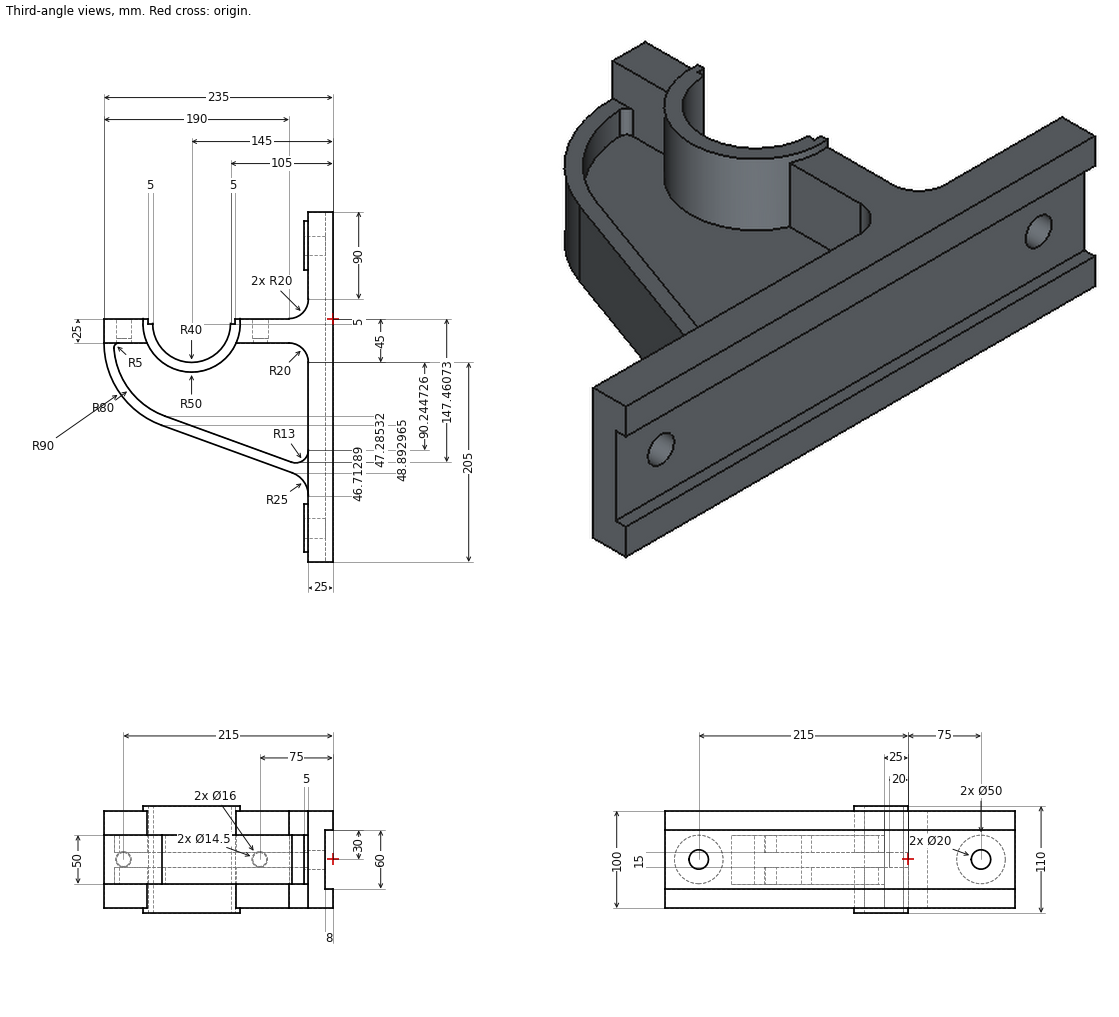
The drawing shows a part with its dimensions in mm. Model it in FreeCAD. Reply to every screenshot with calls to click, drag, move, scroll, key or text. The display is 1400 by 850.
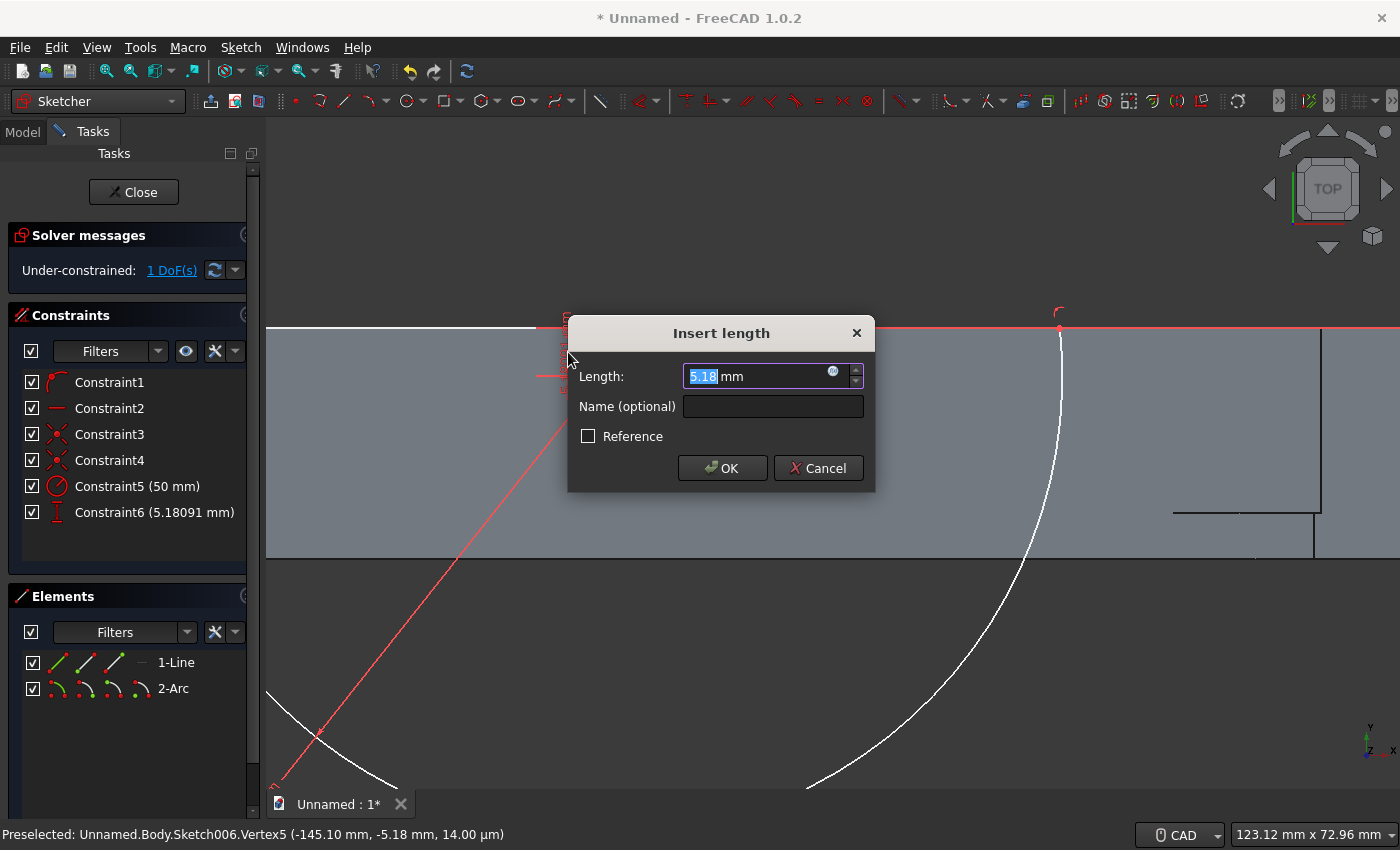
text(5)
key(Return)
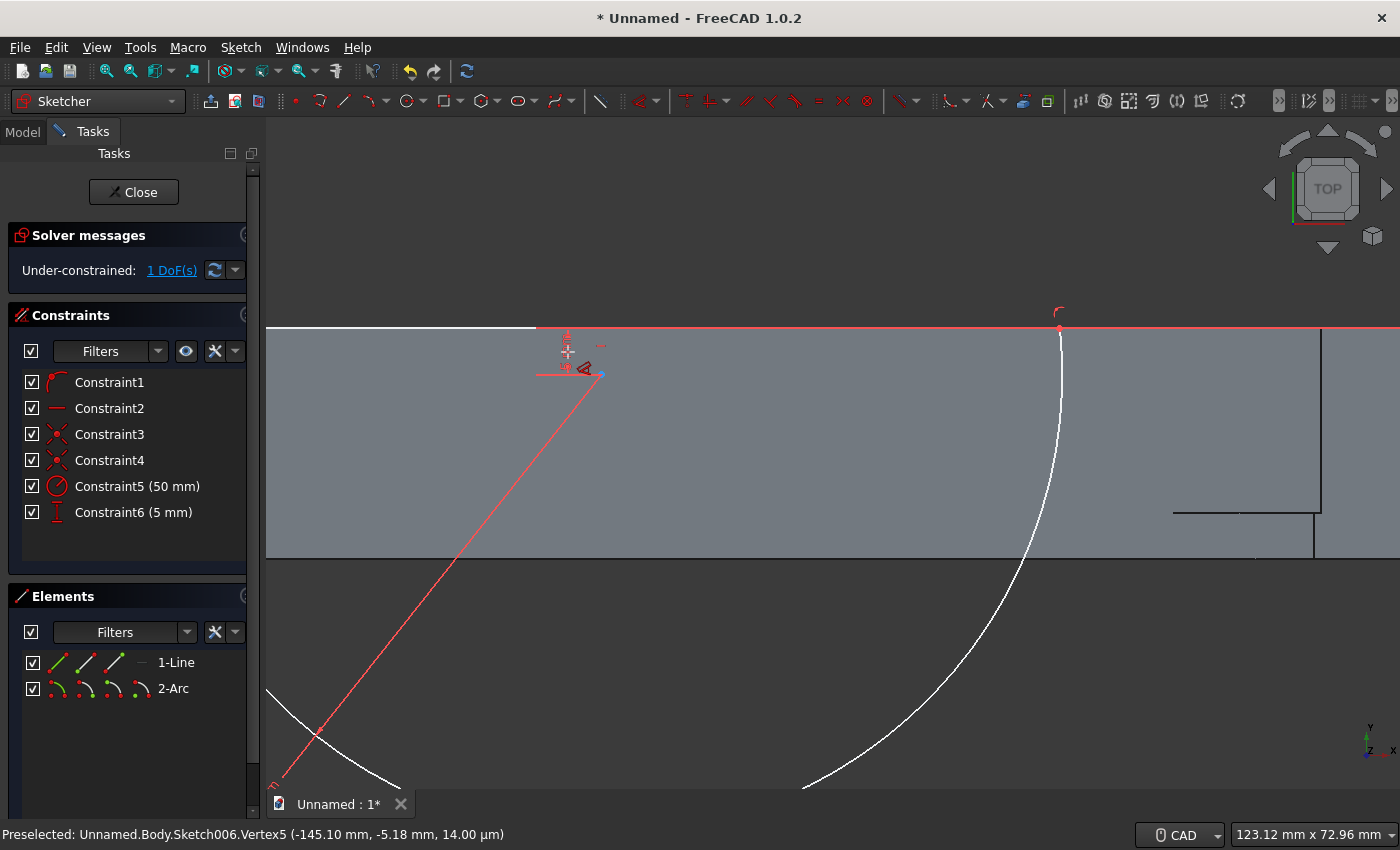
click(602, 375)
click(918, 294)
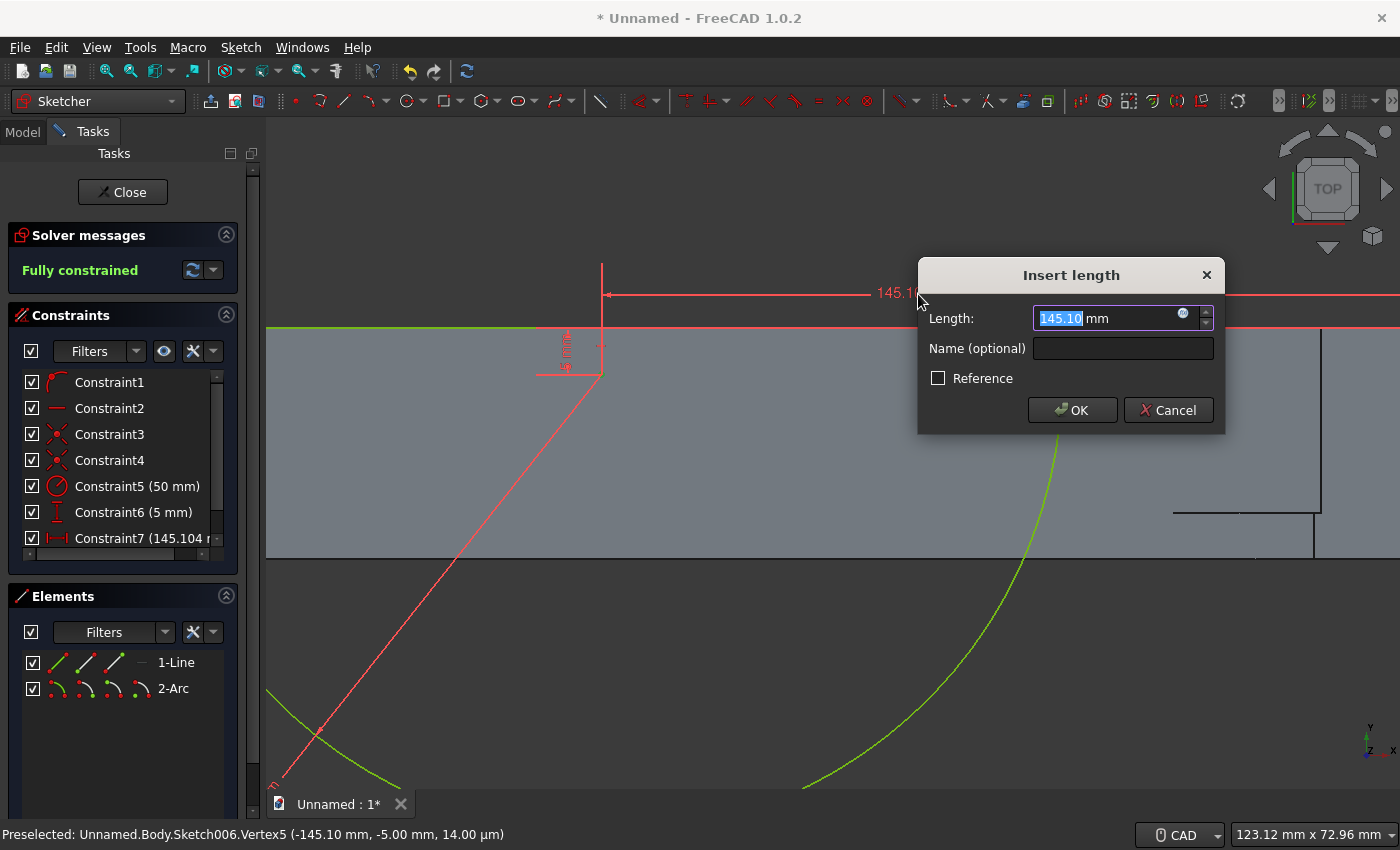
text(145)
key(Return)
key(Escape)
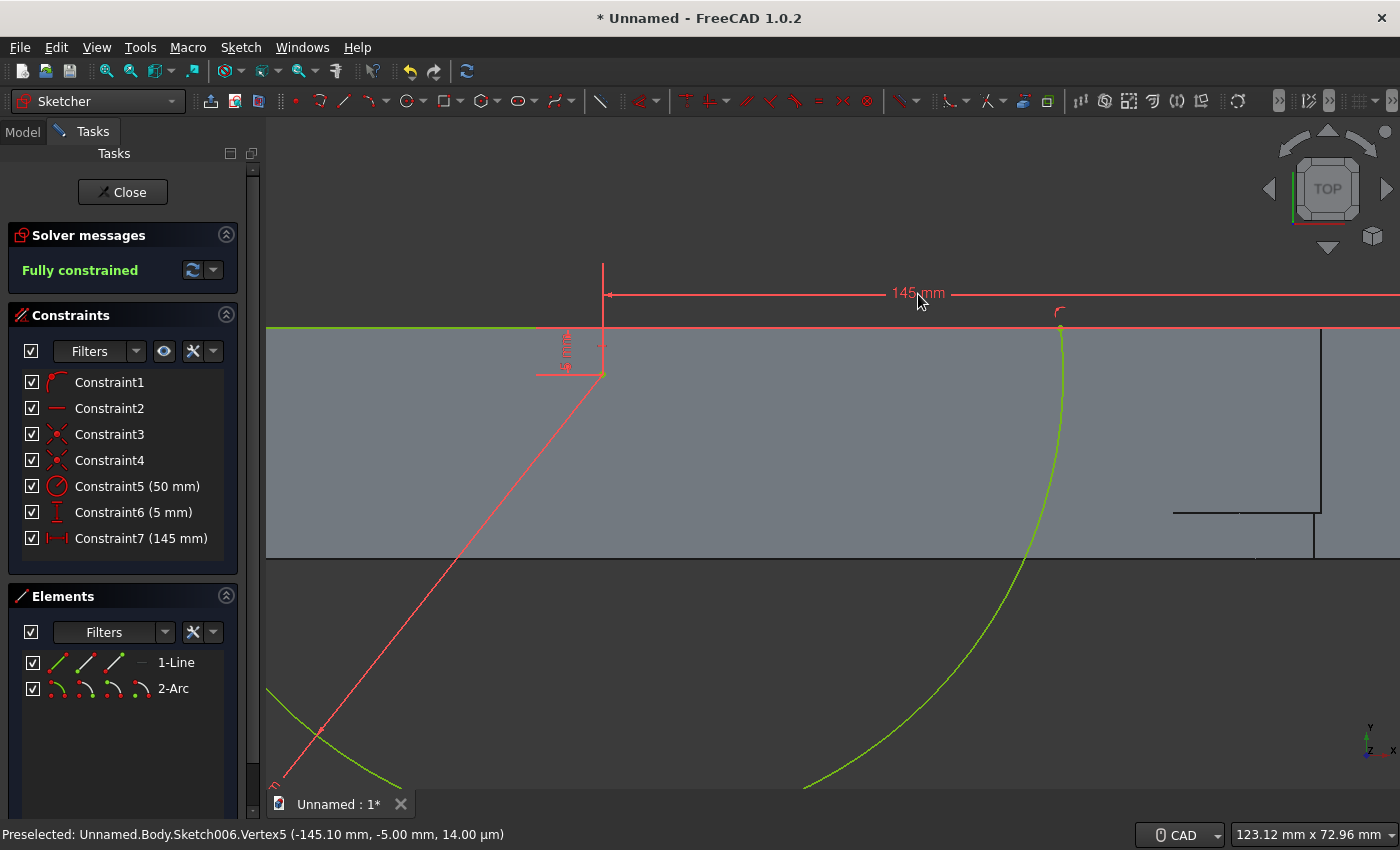
click(123, 192)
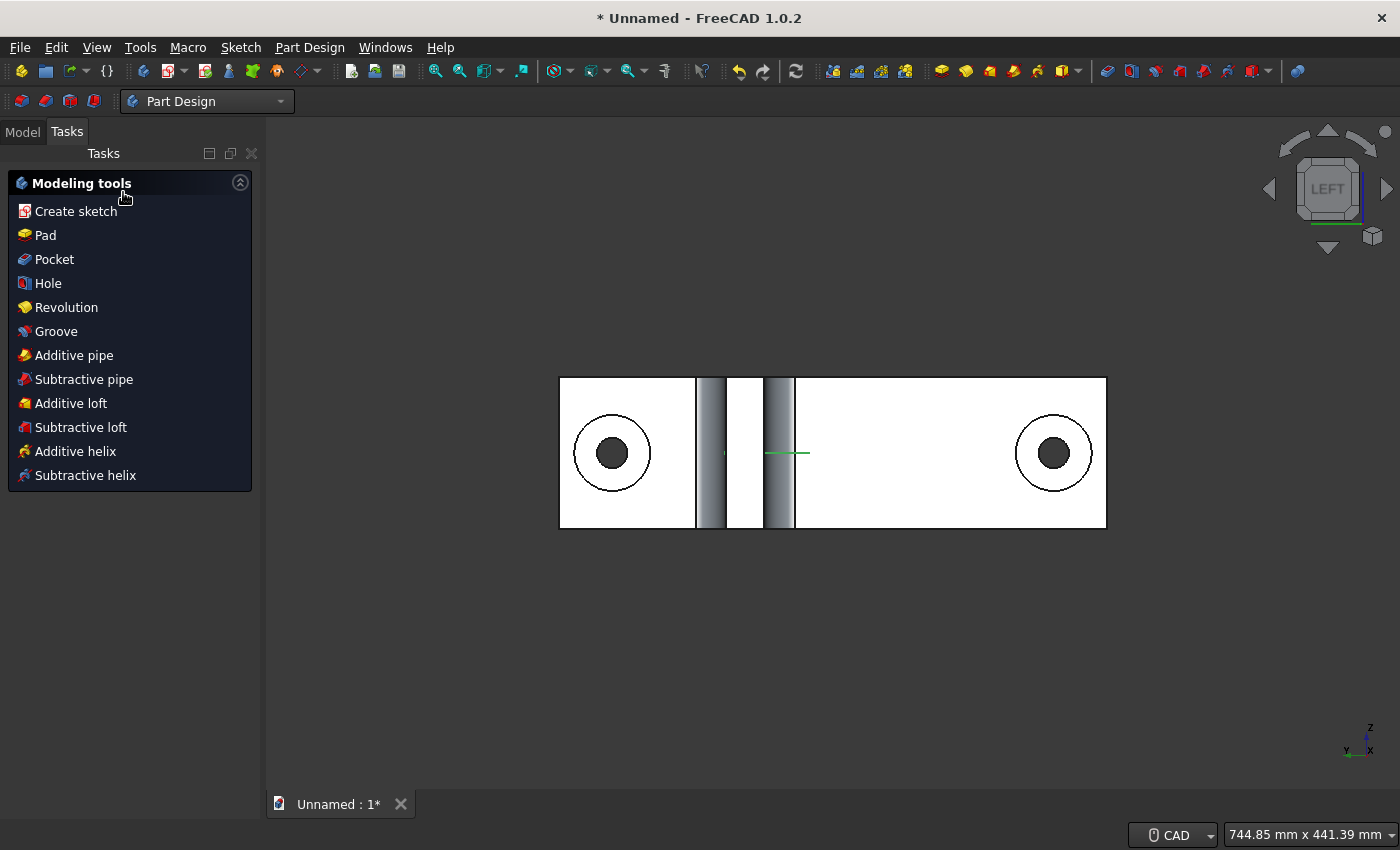
click(942, 72)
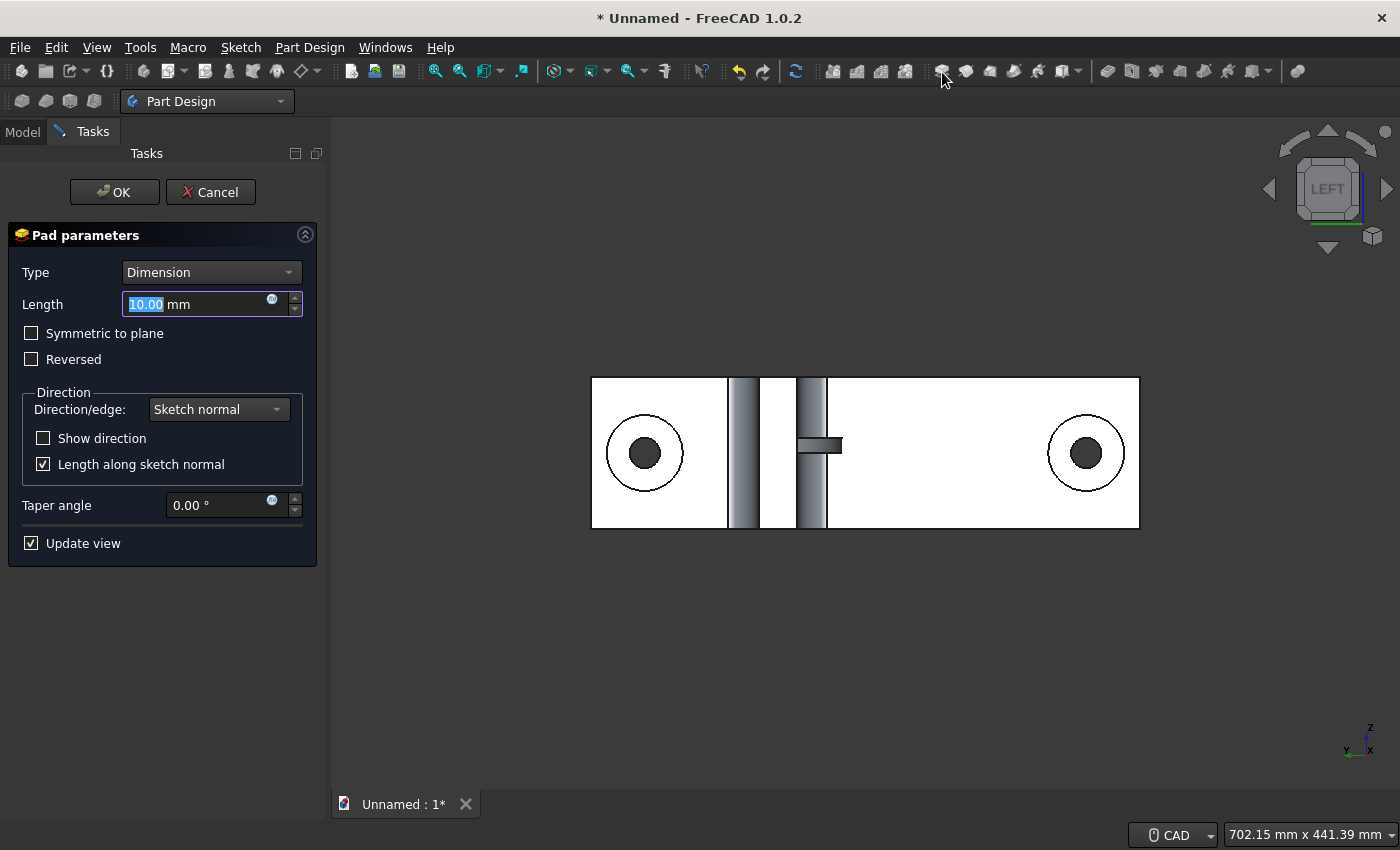
text(110)
key(Tab)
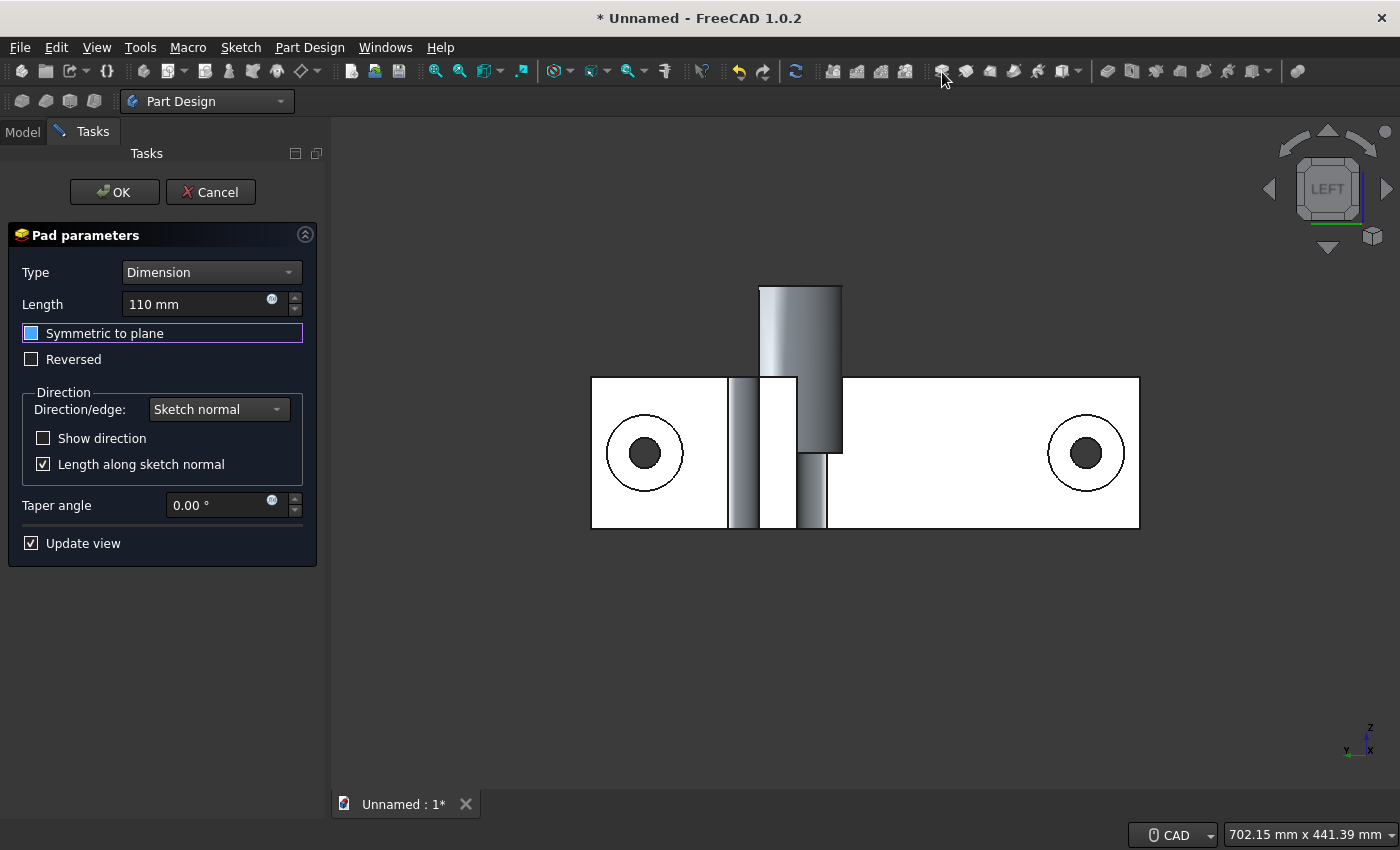
click(30, 333)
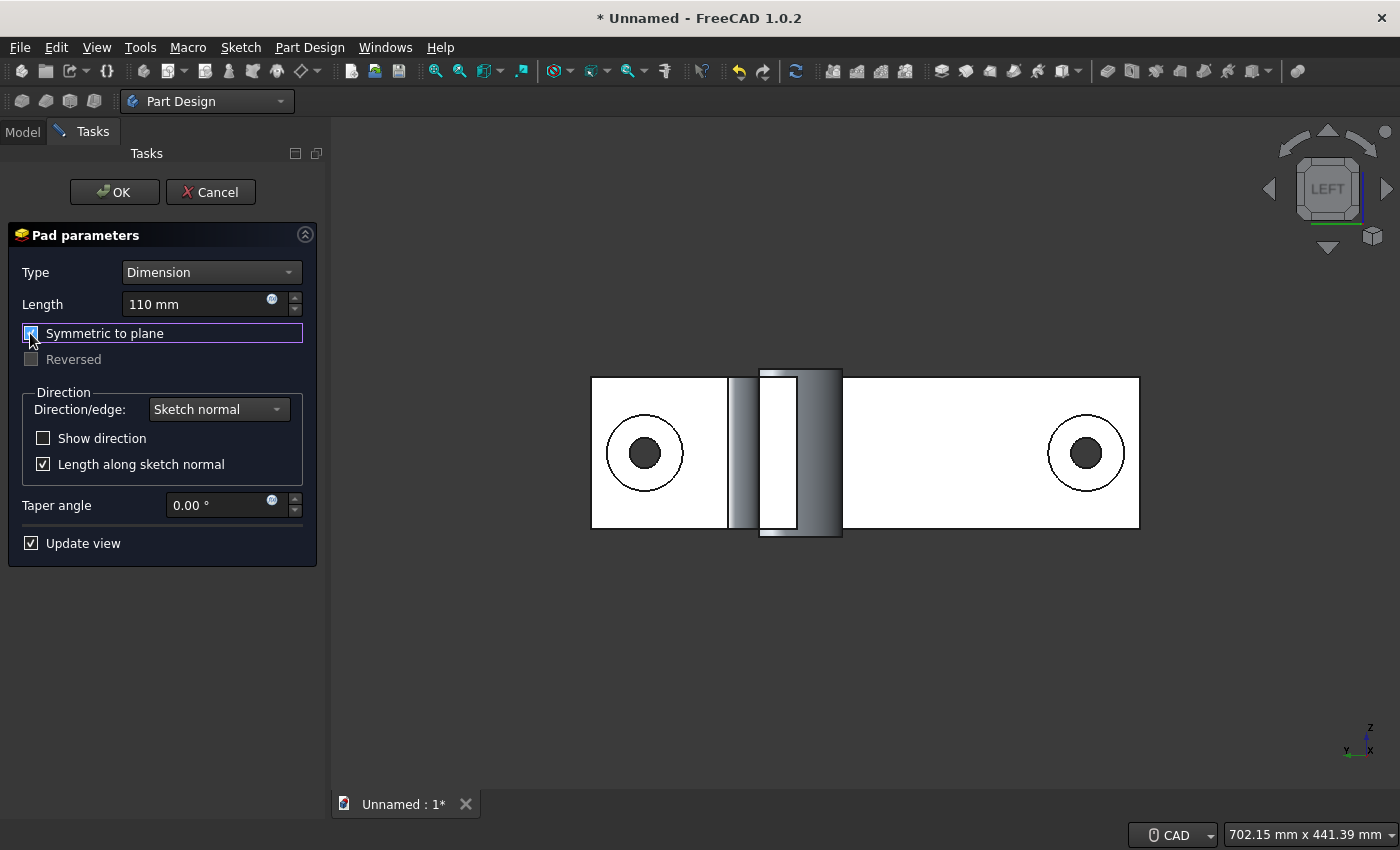
click(115, 192)